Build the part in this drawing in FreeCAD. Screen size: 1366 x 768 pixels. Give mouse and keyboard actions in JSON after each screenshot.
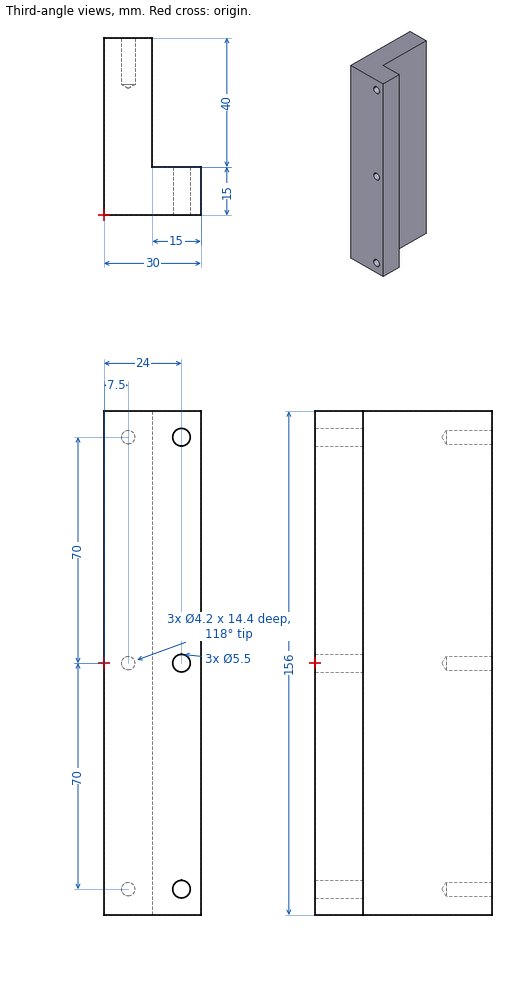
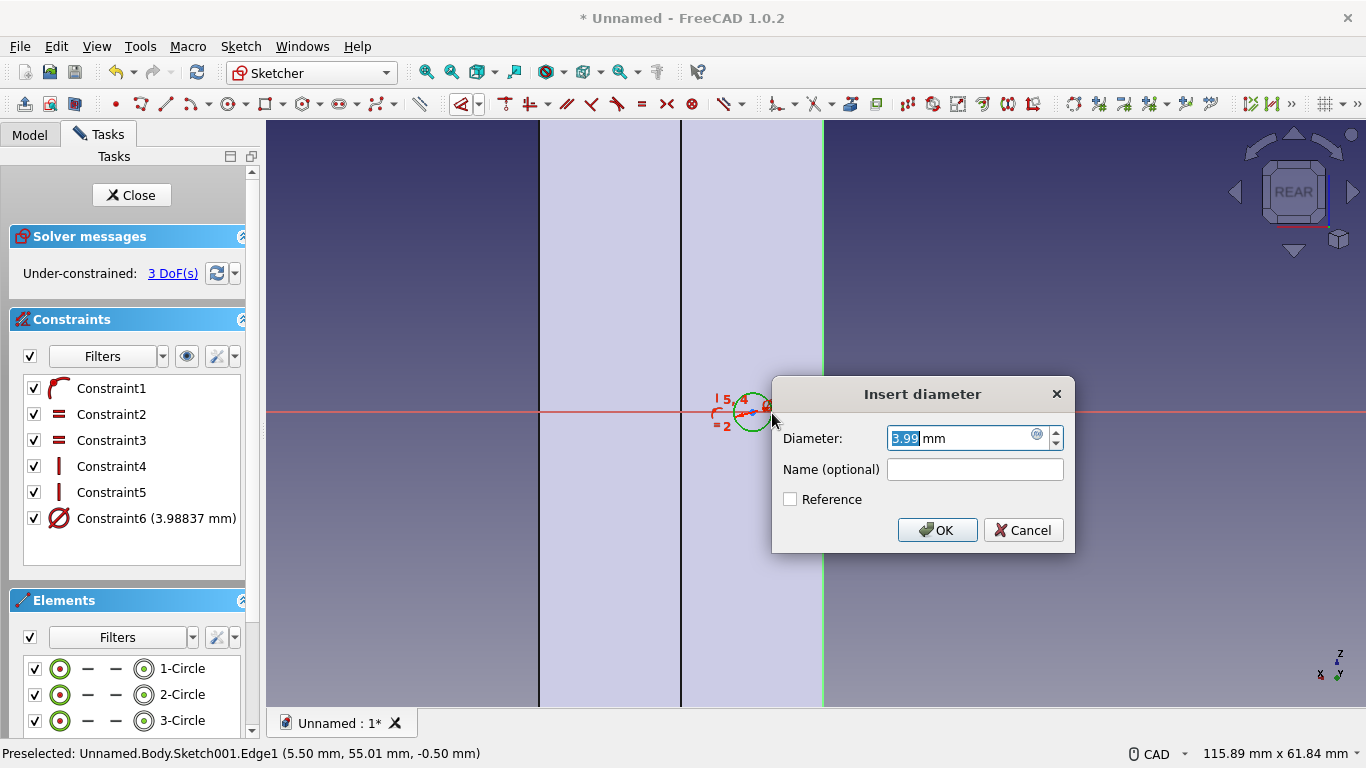
{"action": "type", "text": "4.2"}
{"action": "key", "text": "Return"}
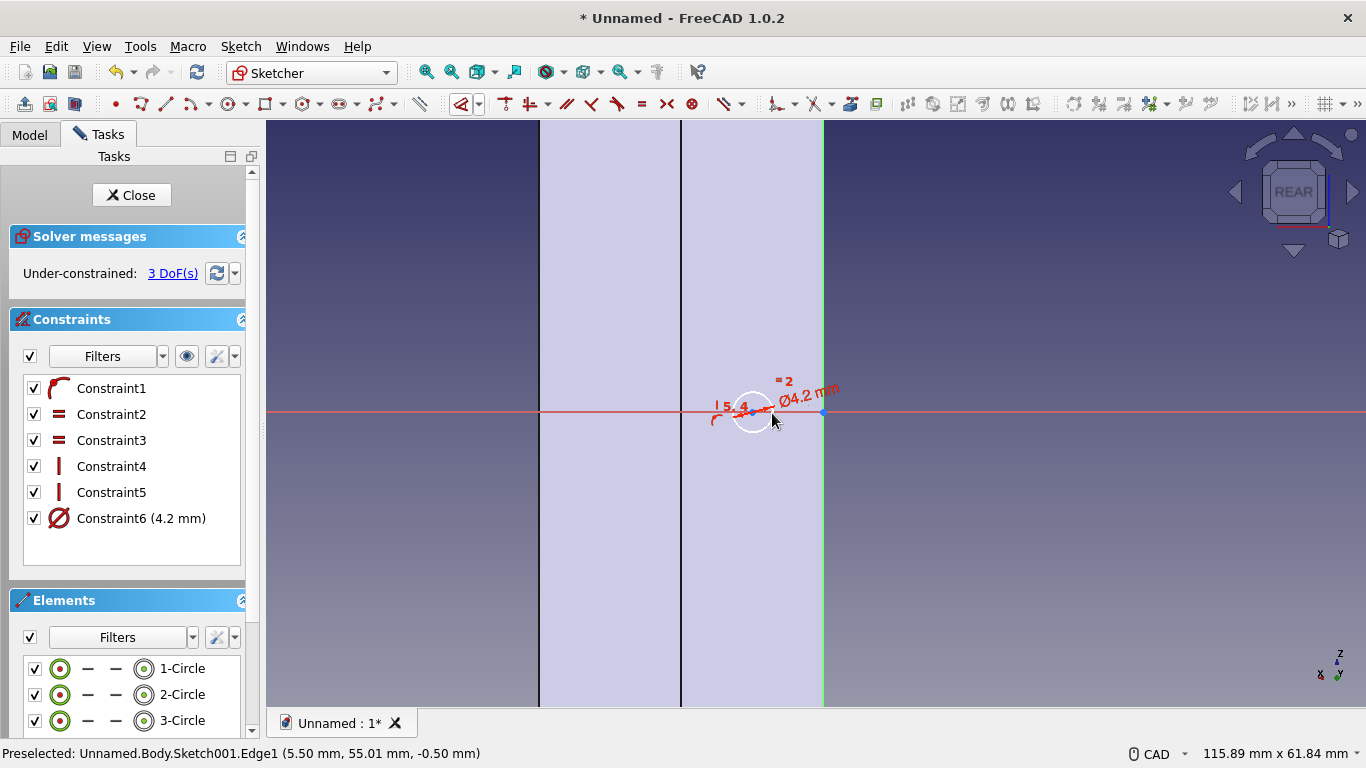
{"action": "scroll", "coordinate": [734, 414], "scroll_direction": "down", "scroll_amount": 6}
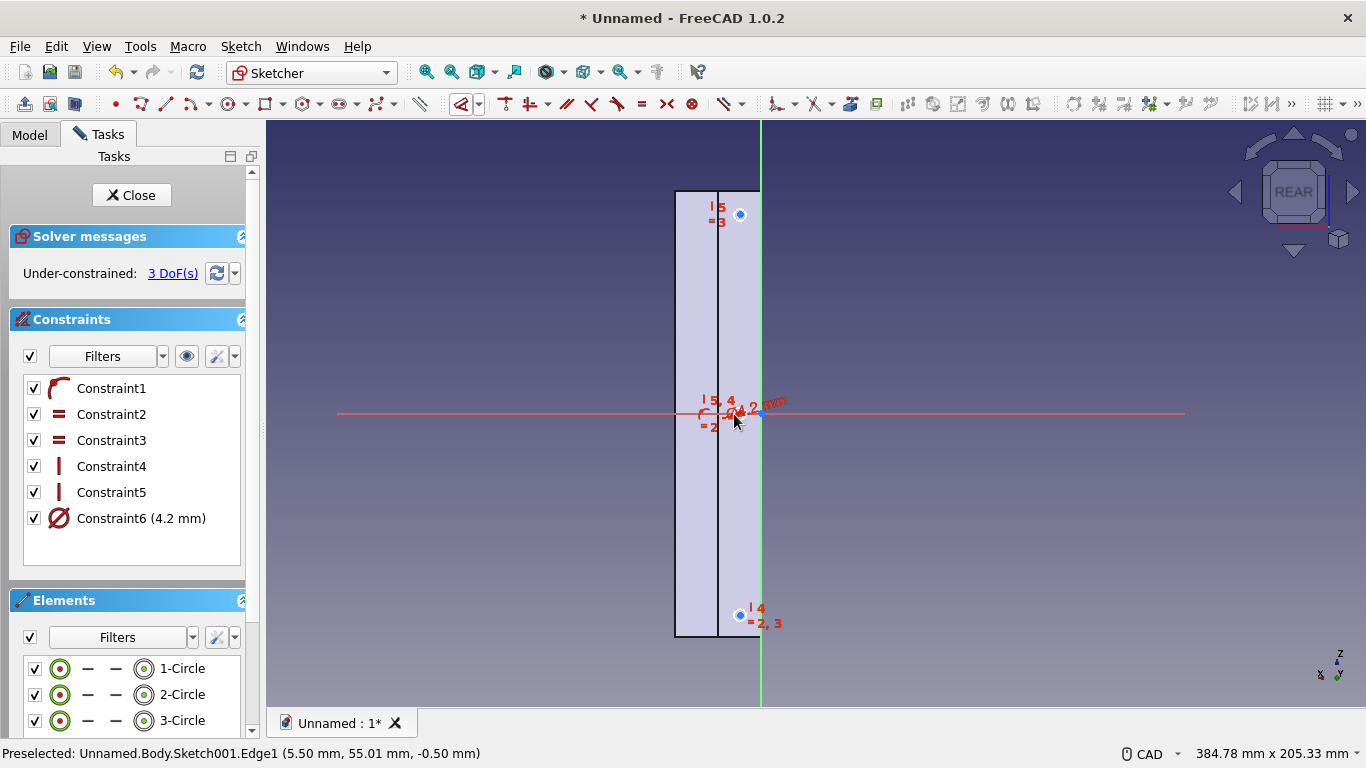
{"action": "left_click", "coordinate": [740, 615]}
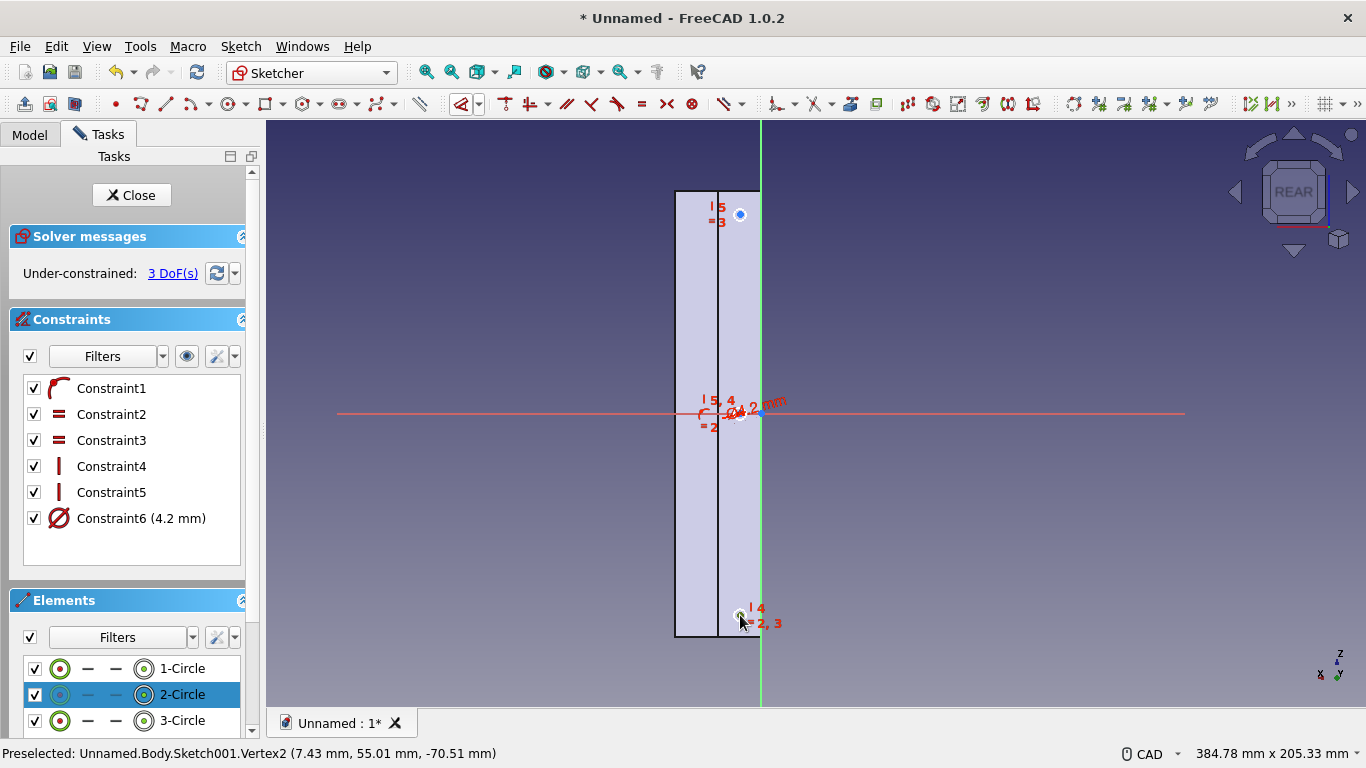
{"action": "key", "text": "i"}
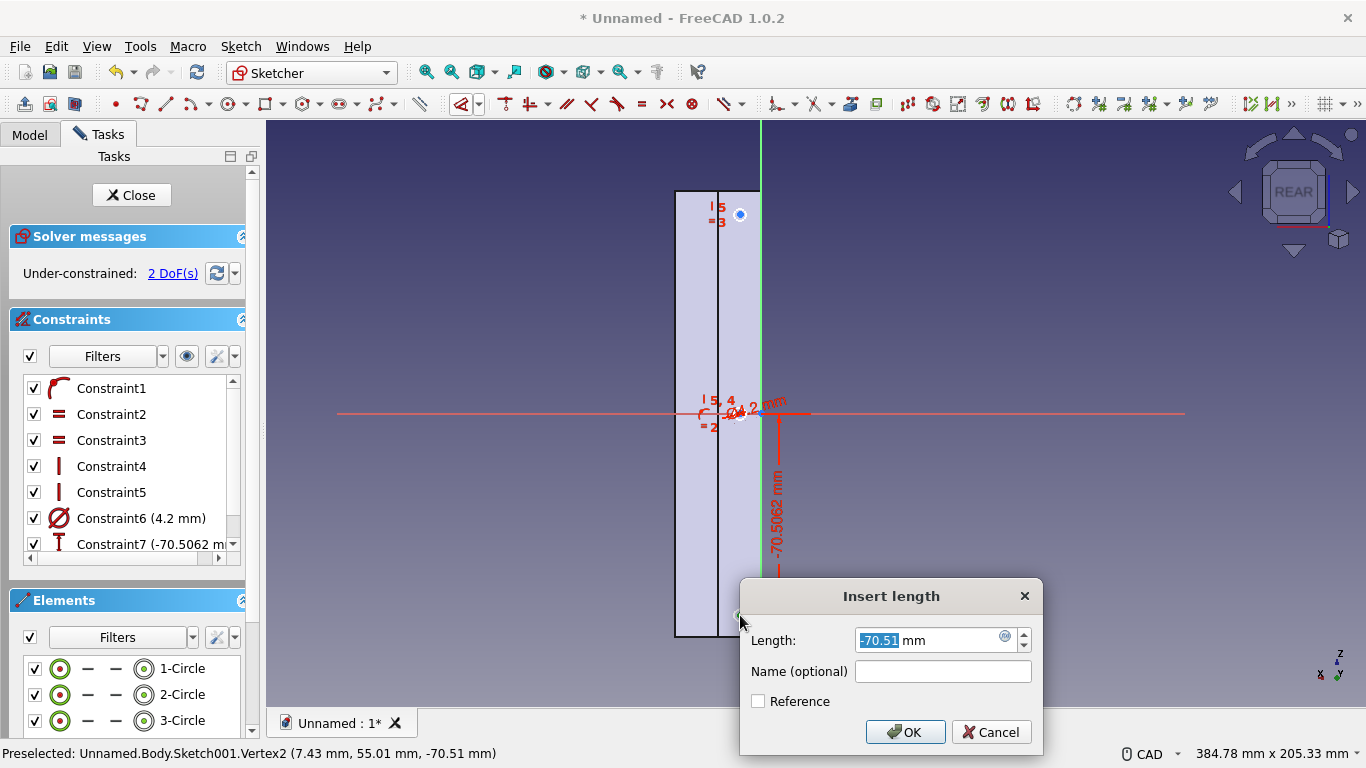
{"action": "type", "text": "-70"}
{"action": "key", "text": "Return"}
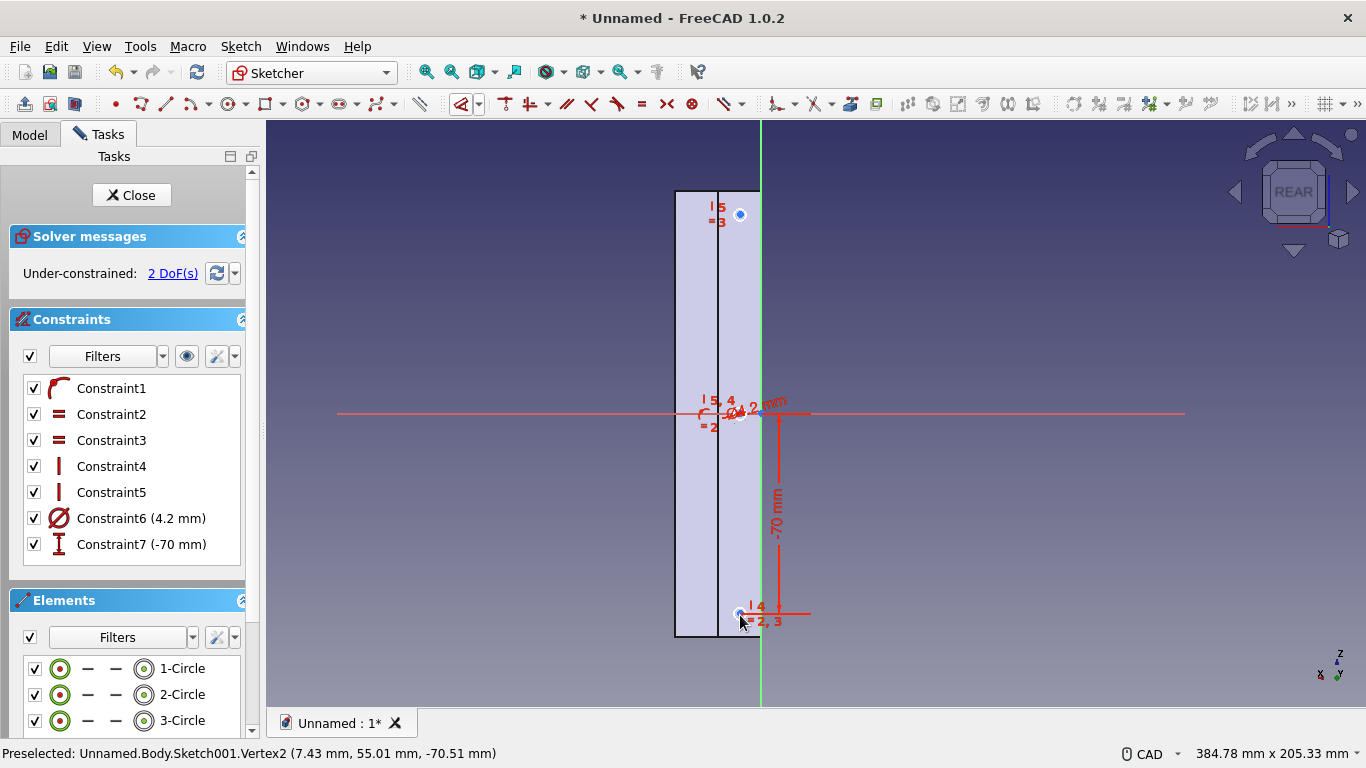
{"action": "left_click", "coordinate": [740, 215]}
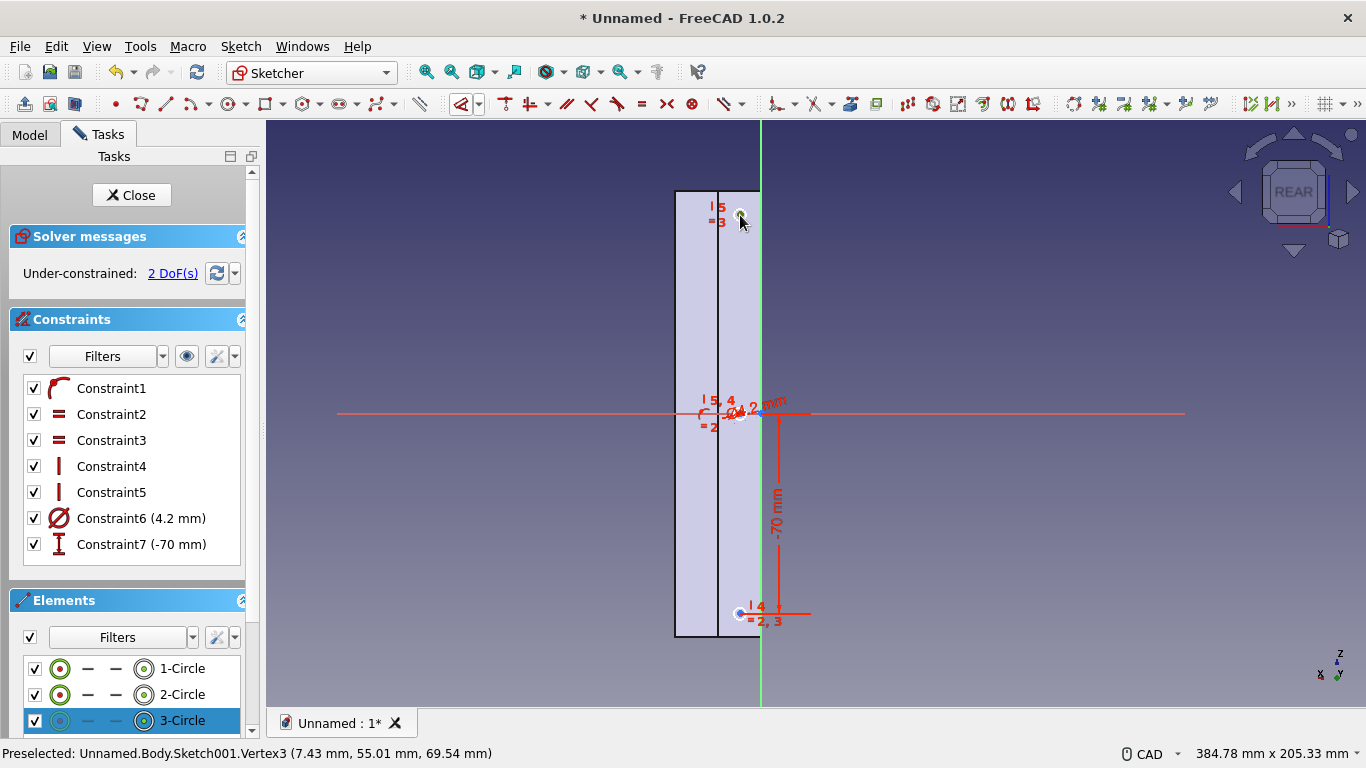
{"action": "key", "text": "i"}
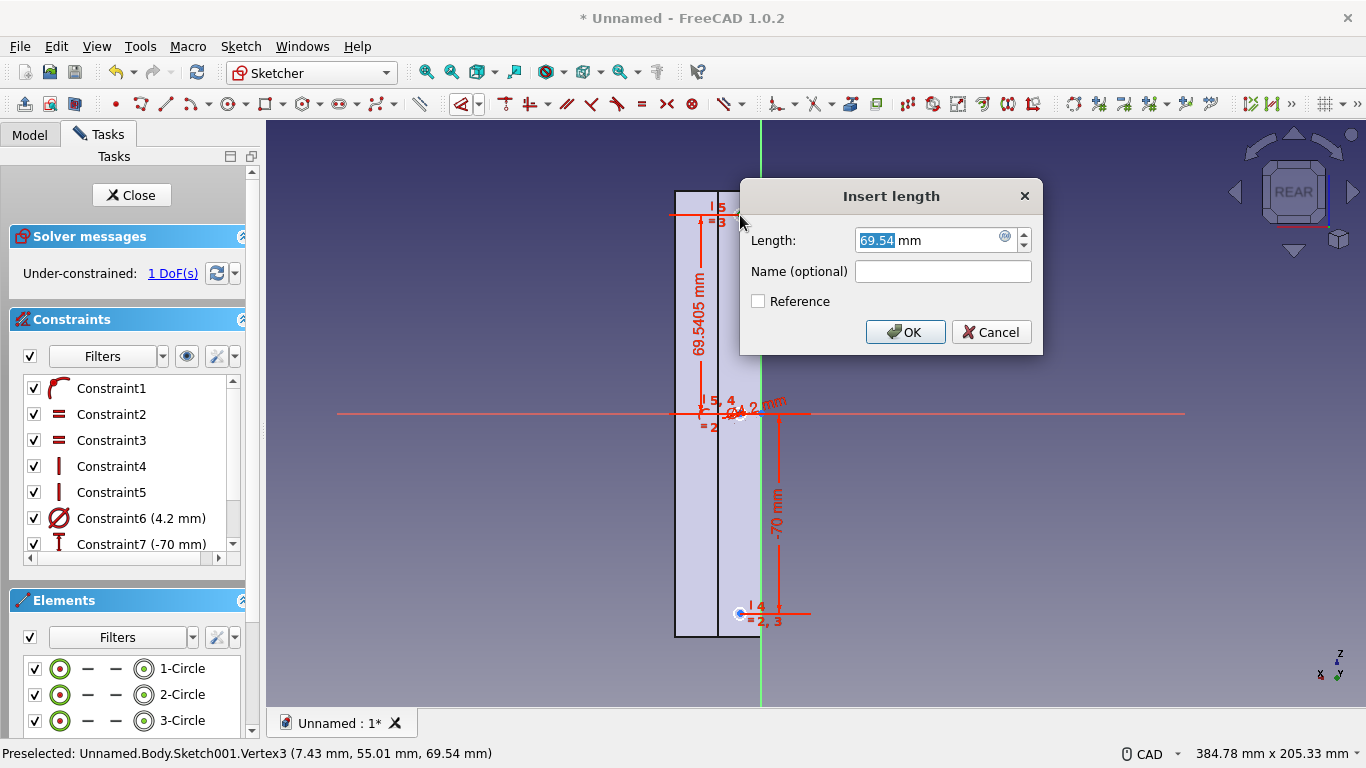
{"action": "type", "text": "70"}
{"action": "key", "text": "Return"}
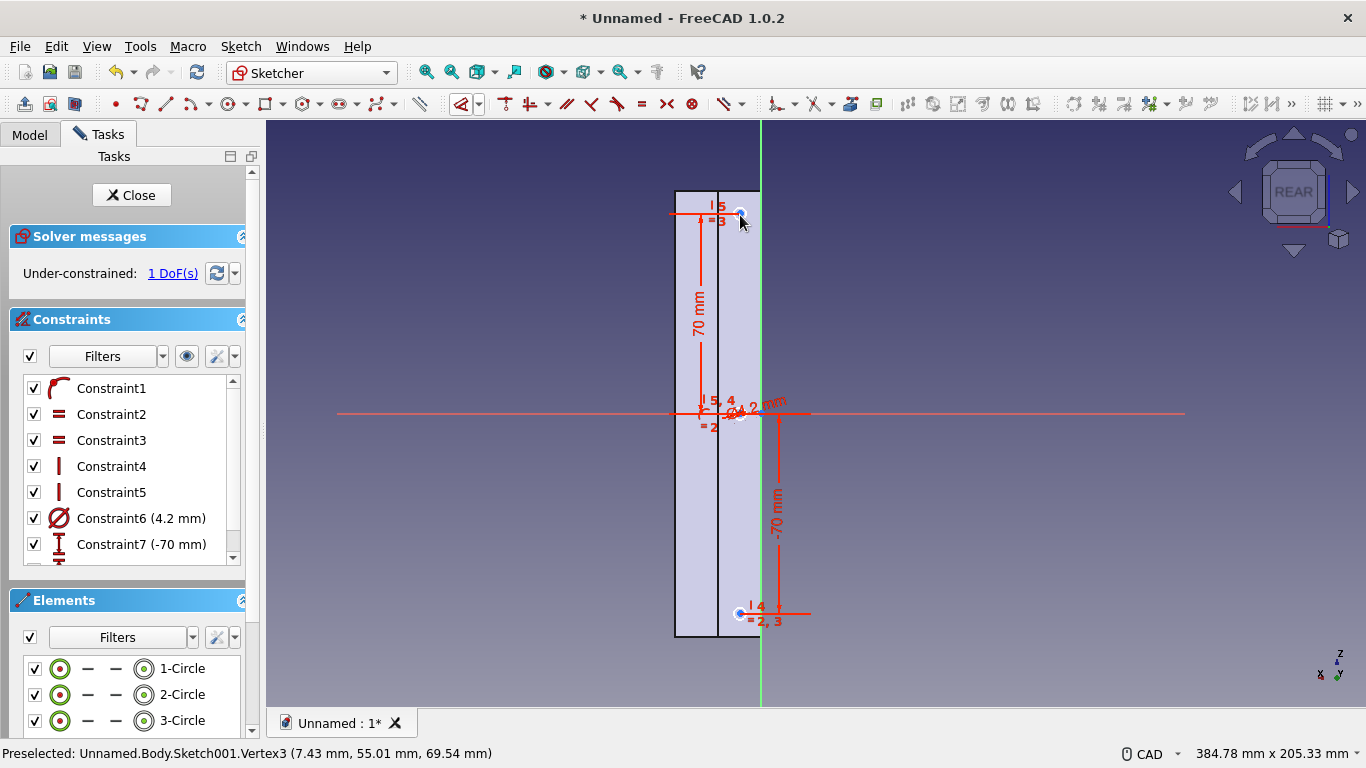
{"action": "scroll", "coordinate": [740, 414], "scroll_direction": "up", "scroll_amount": 4}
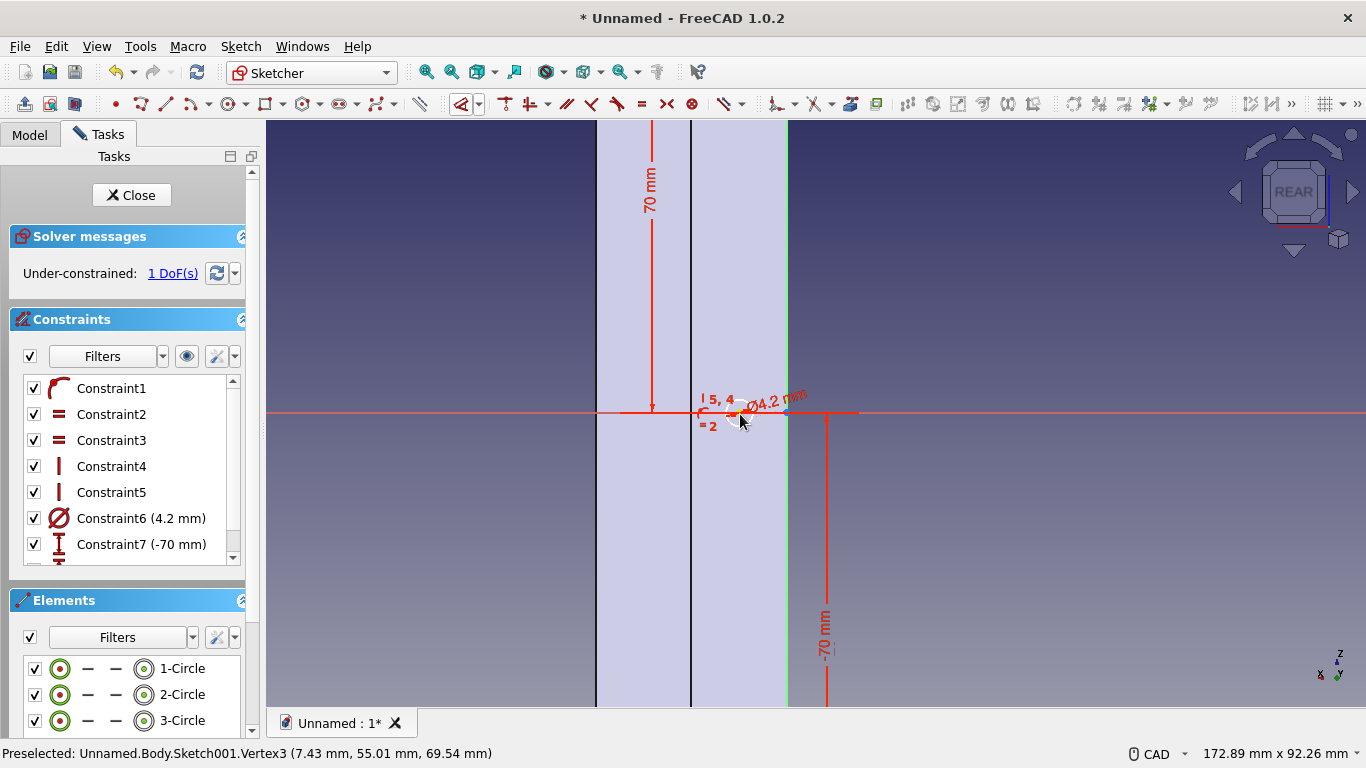
{"action": "left_click", "coordinate": [739, 413]}